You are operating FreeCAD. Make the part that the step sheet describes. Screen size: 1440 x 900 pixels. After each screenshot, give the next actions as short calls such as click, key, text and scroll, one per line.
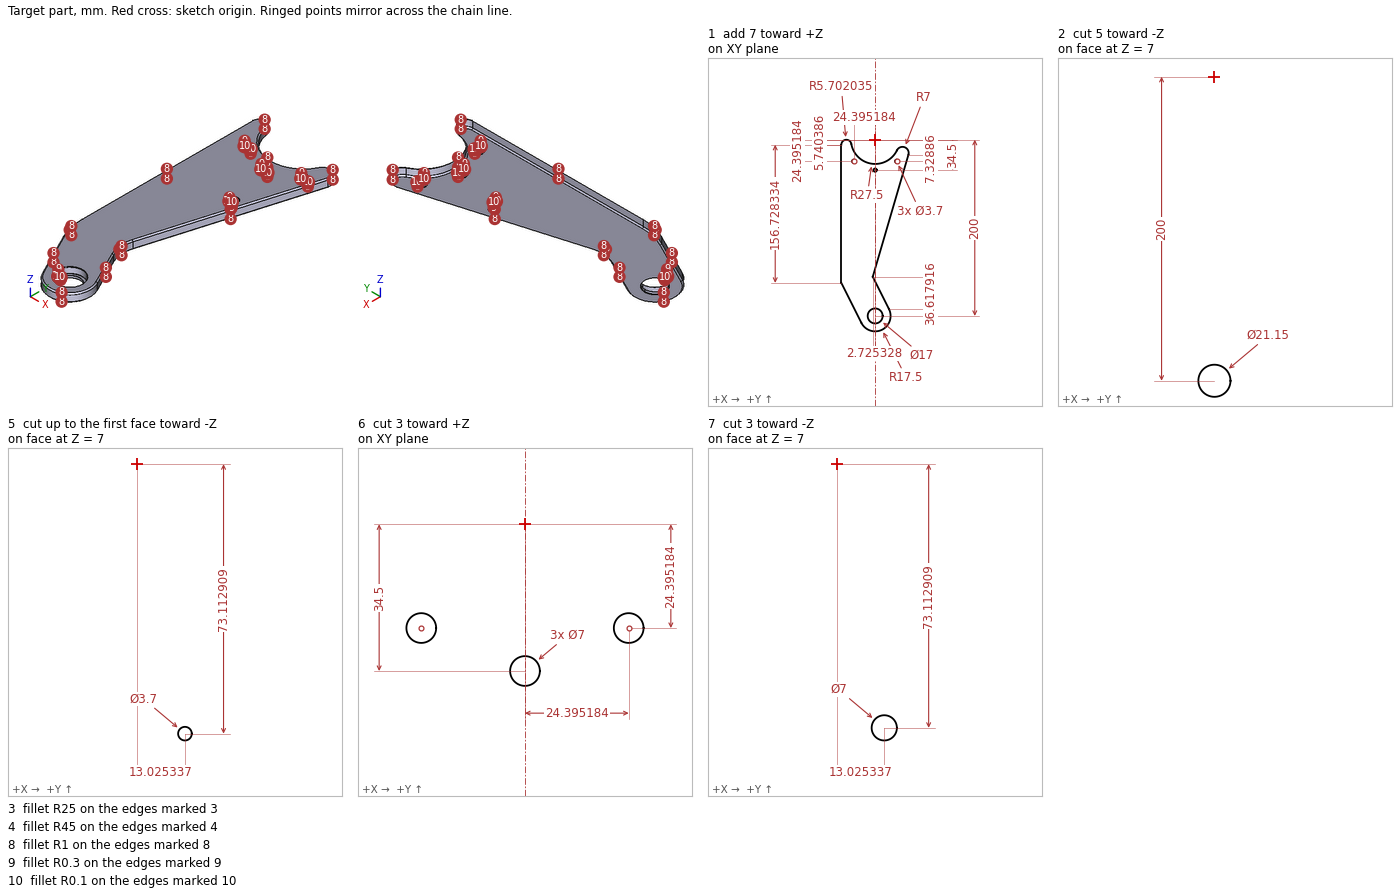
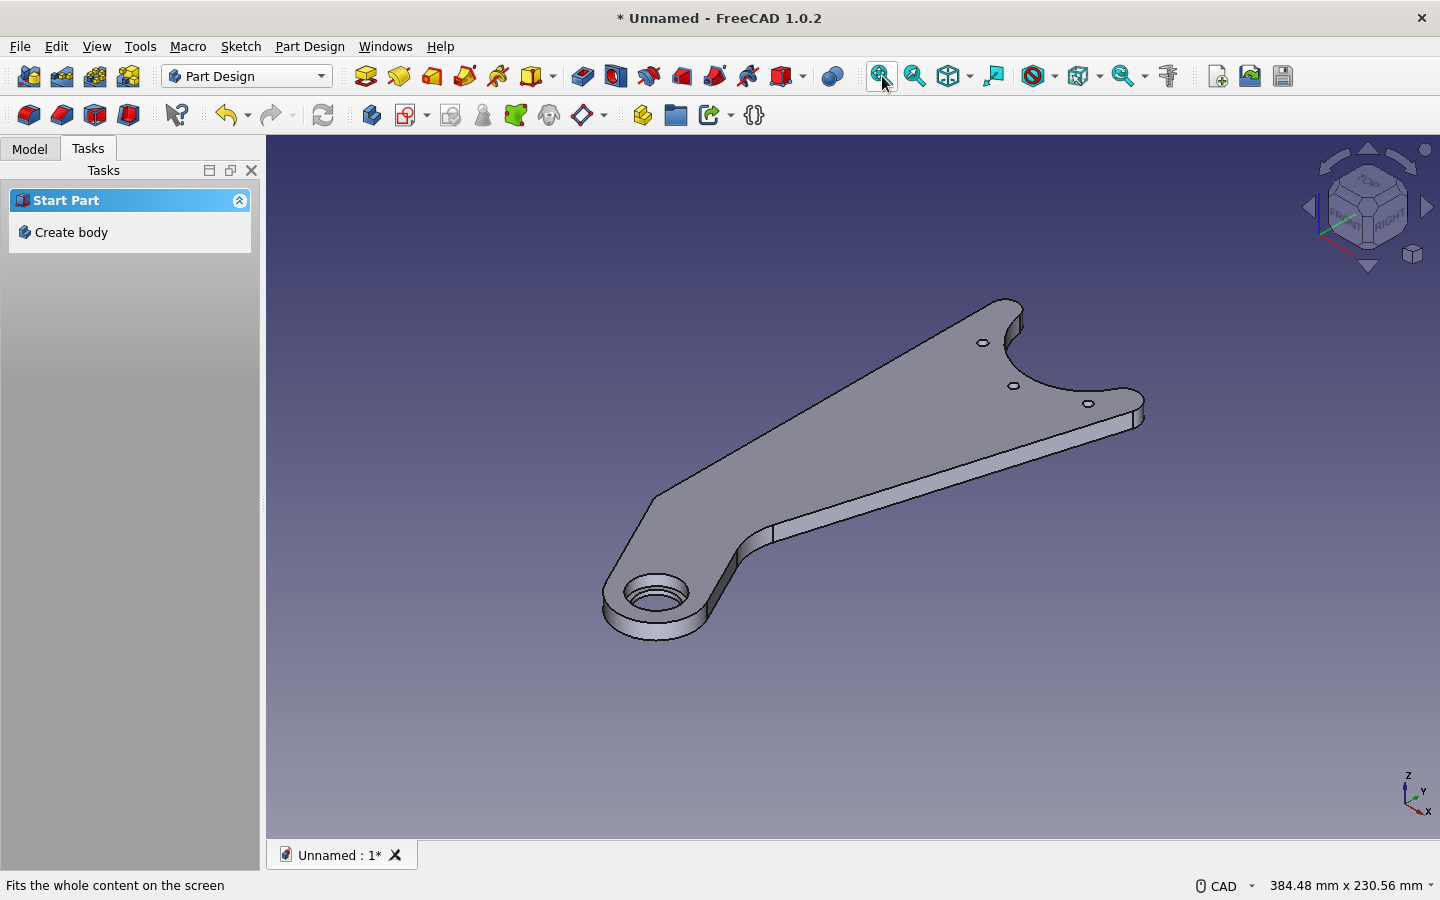
key(2)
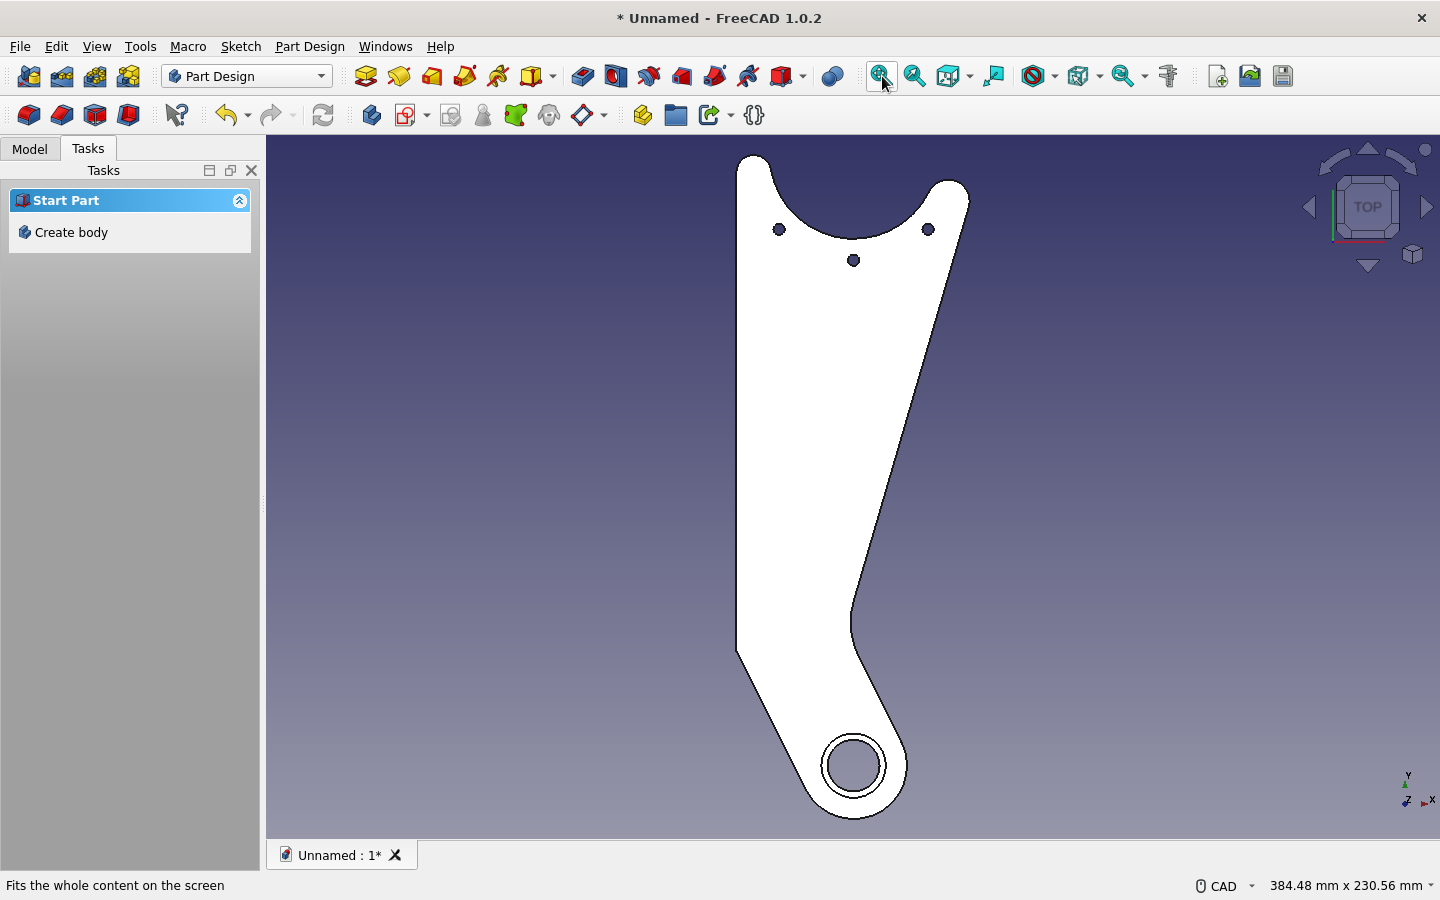
scroll(736, 650, up, 4)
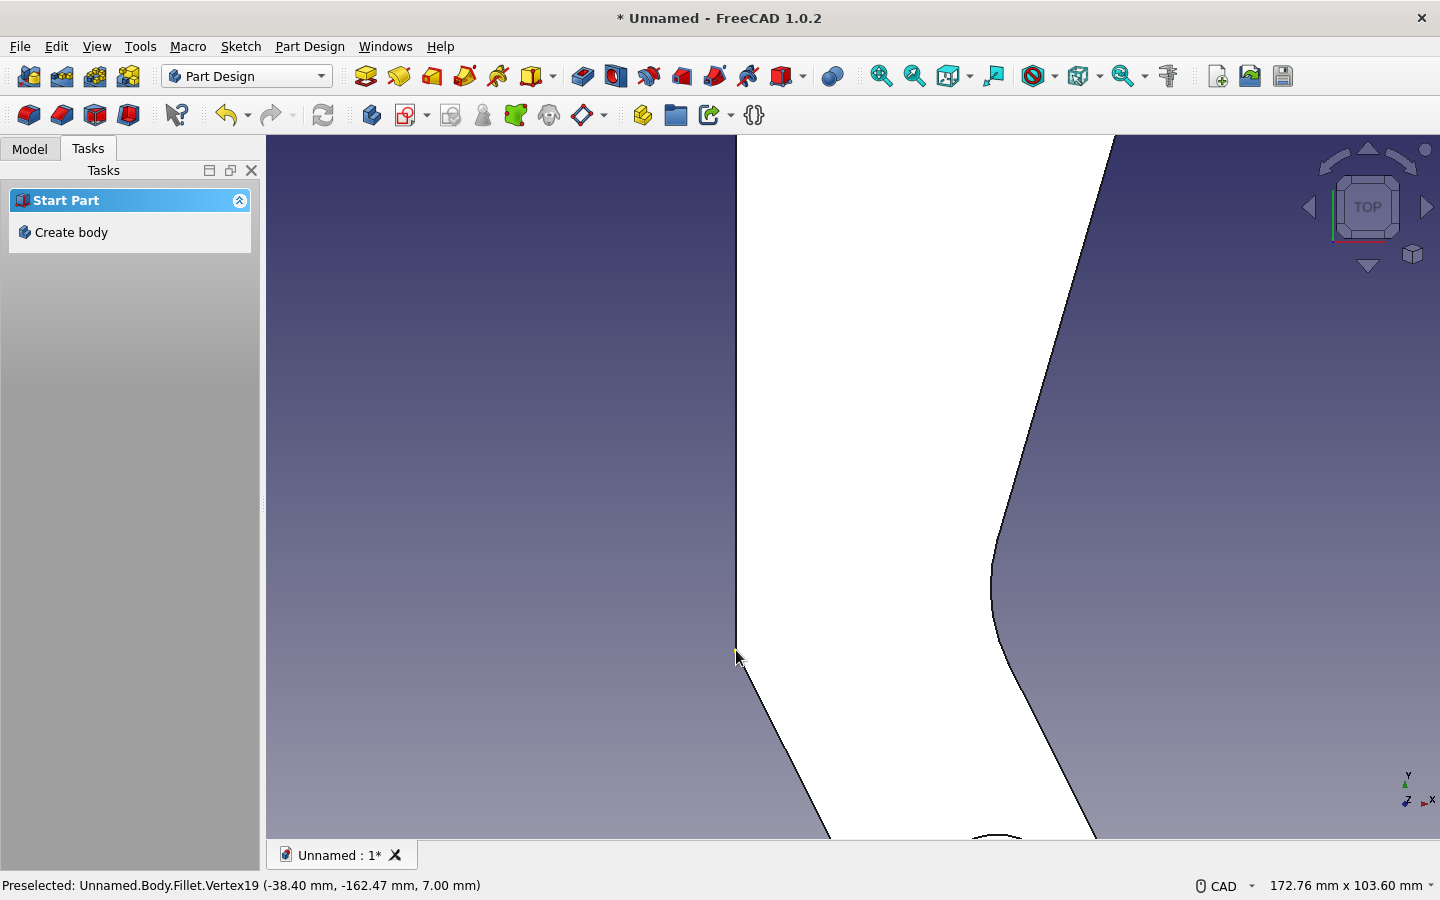
key(v)
key(f)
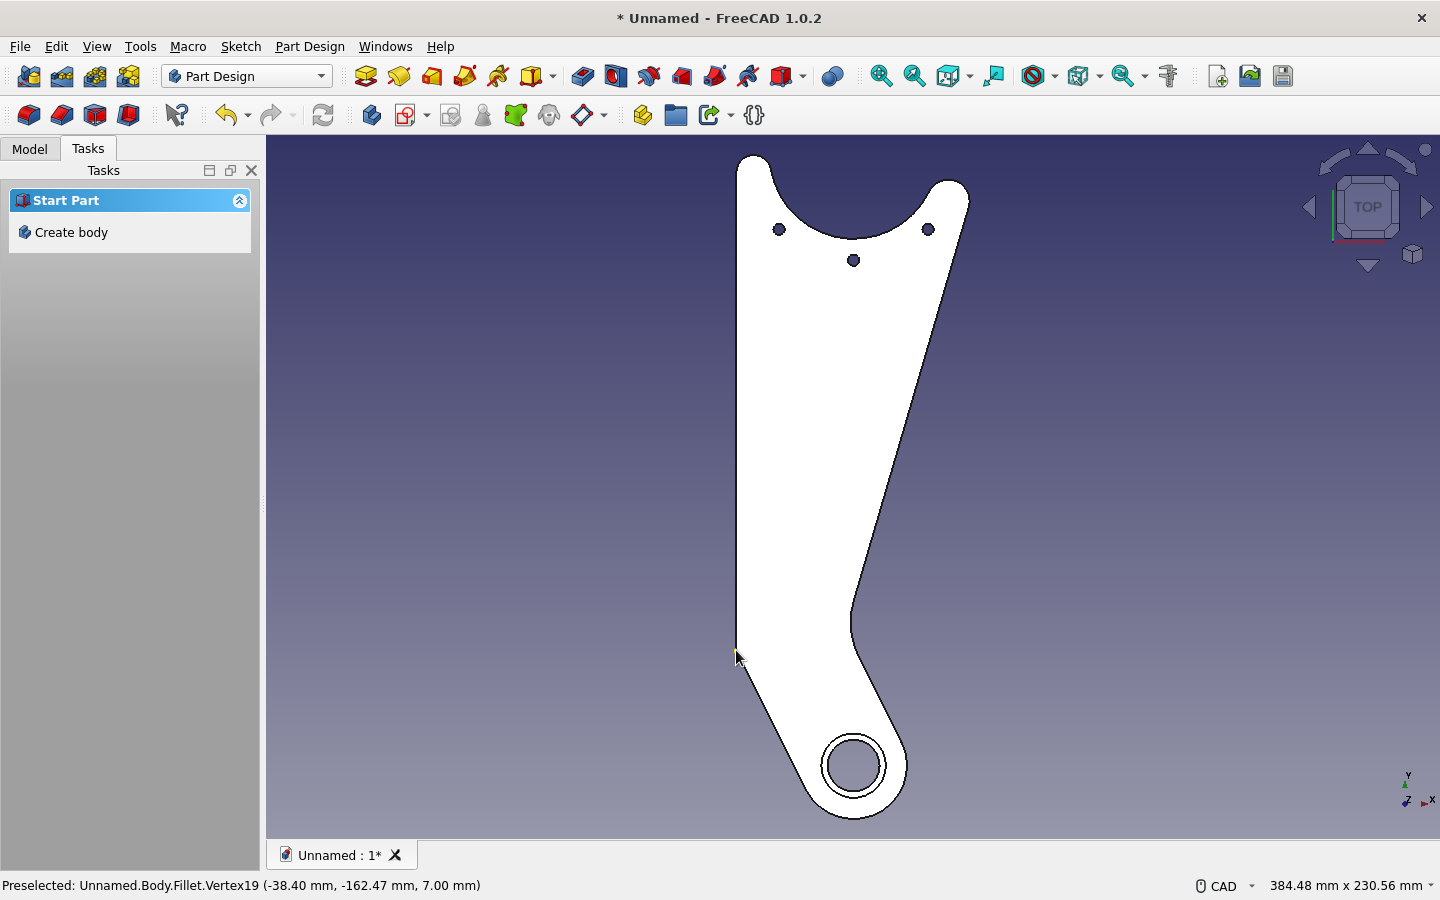
key(0)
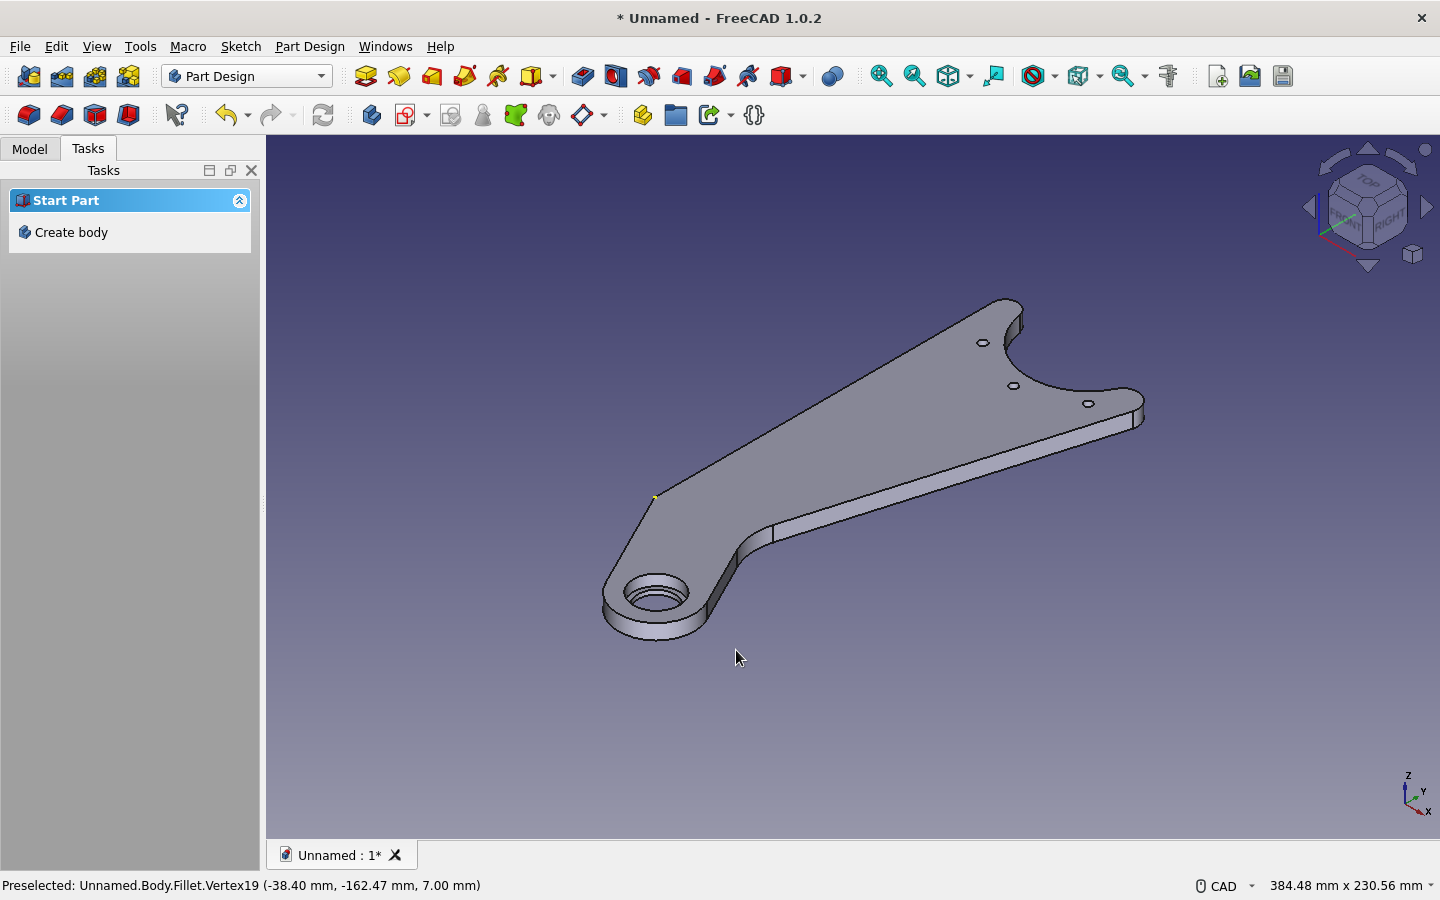
scroll(655, 505, up, 4)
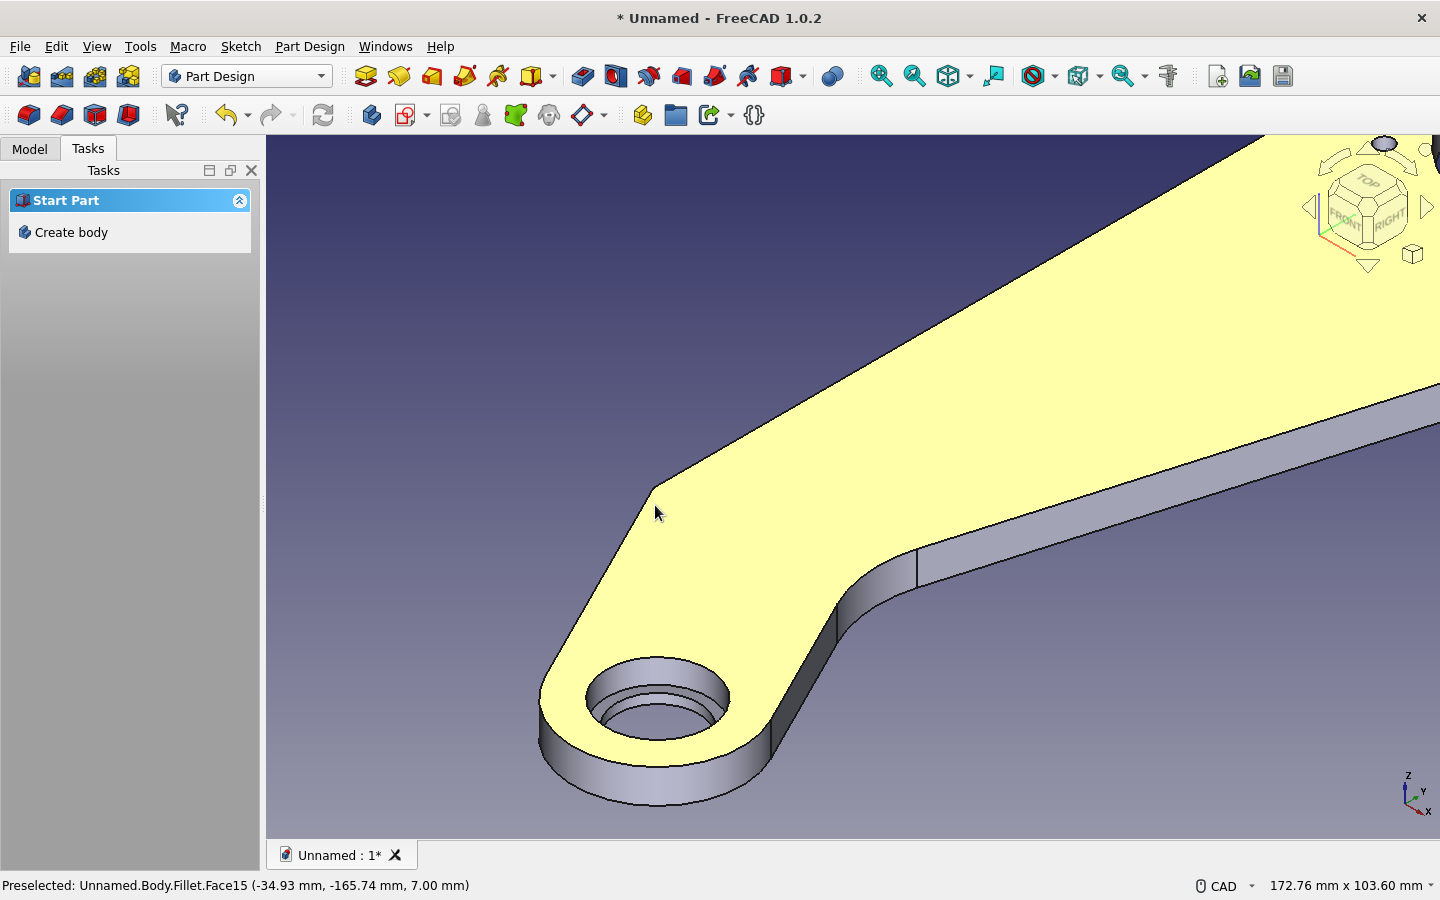
click(882, 76)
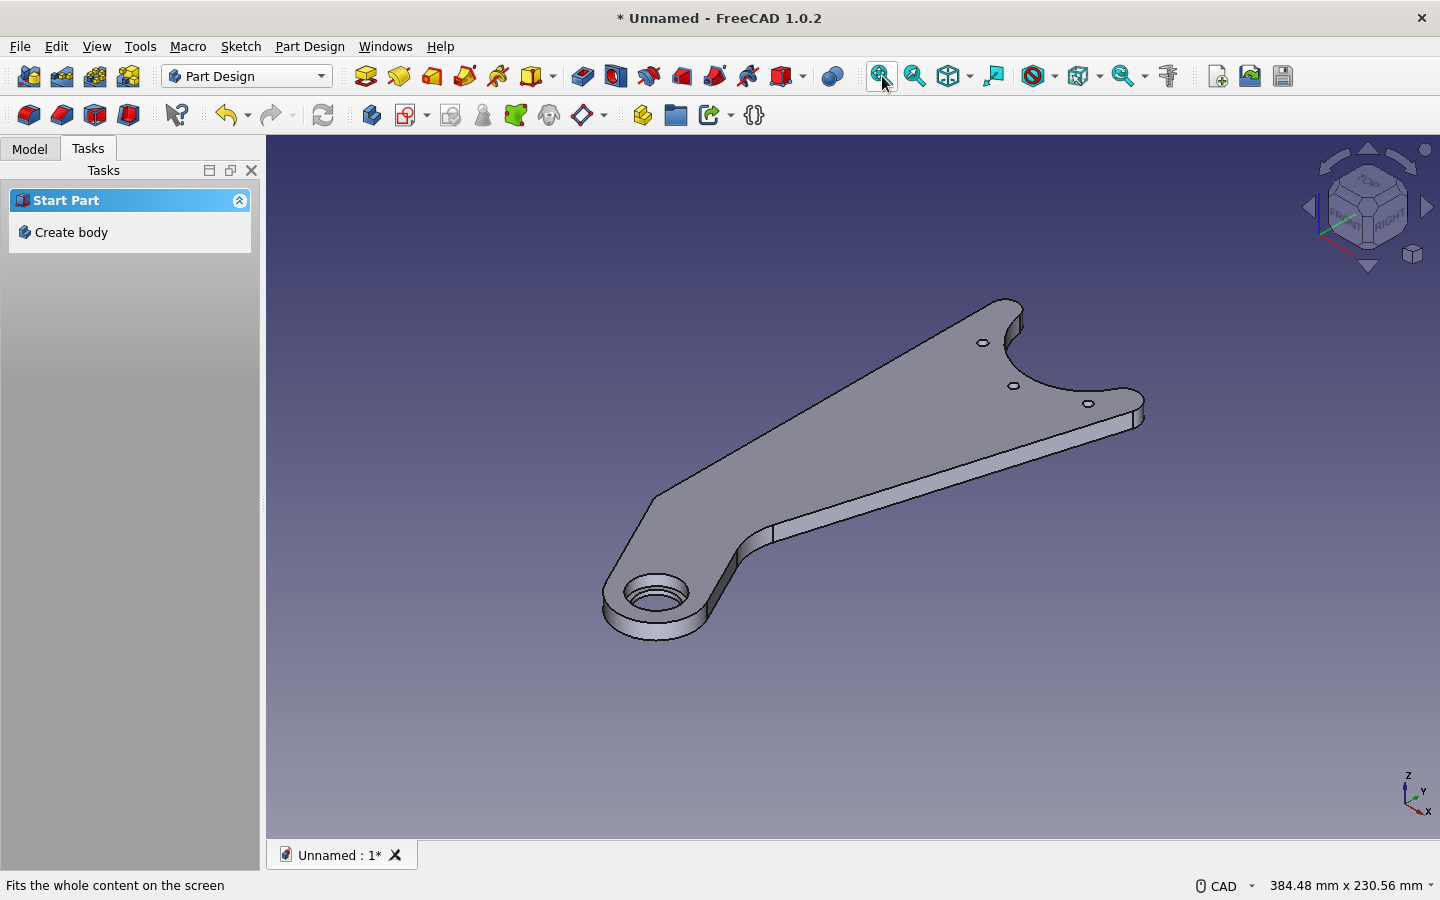
key(1)